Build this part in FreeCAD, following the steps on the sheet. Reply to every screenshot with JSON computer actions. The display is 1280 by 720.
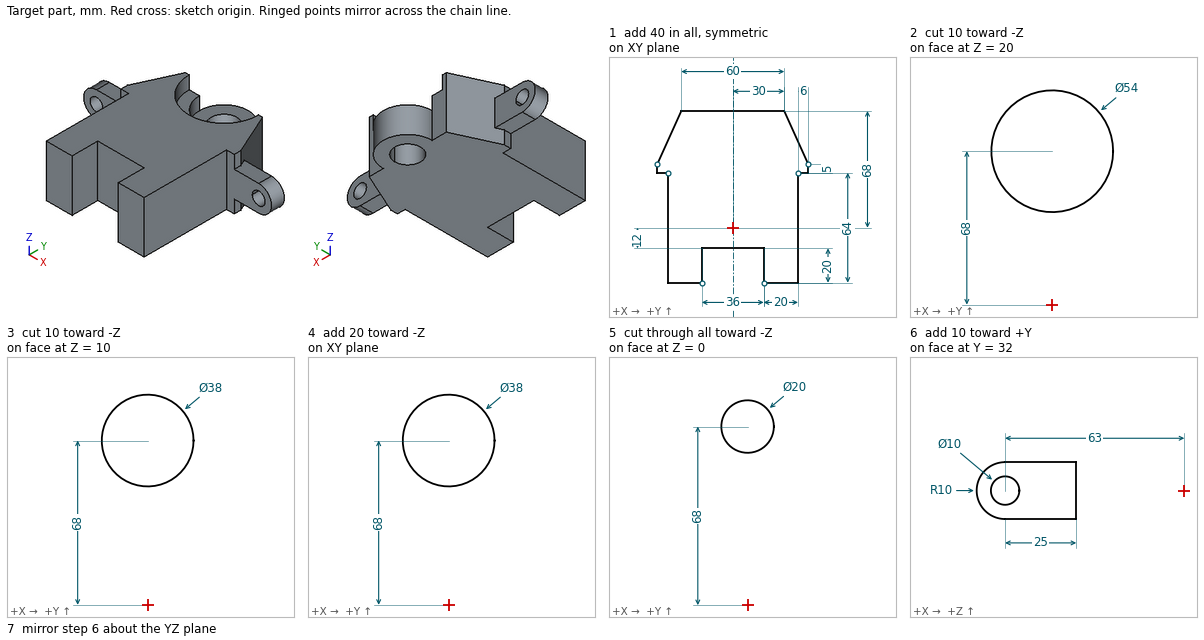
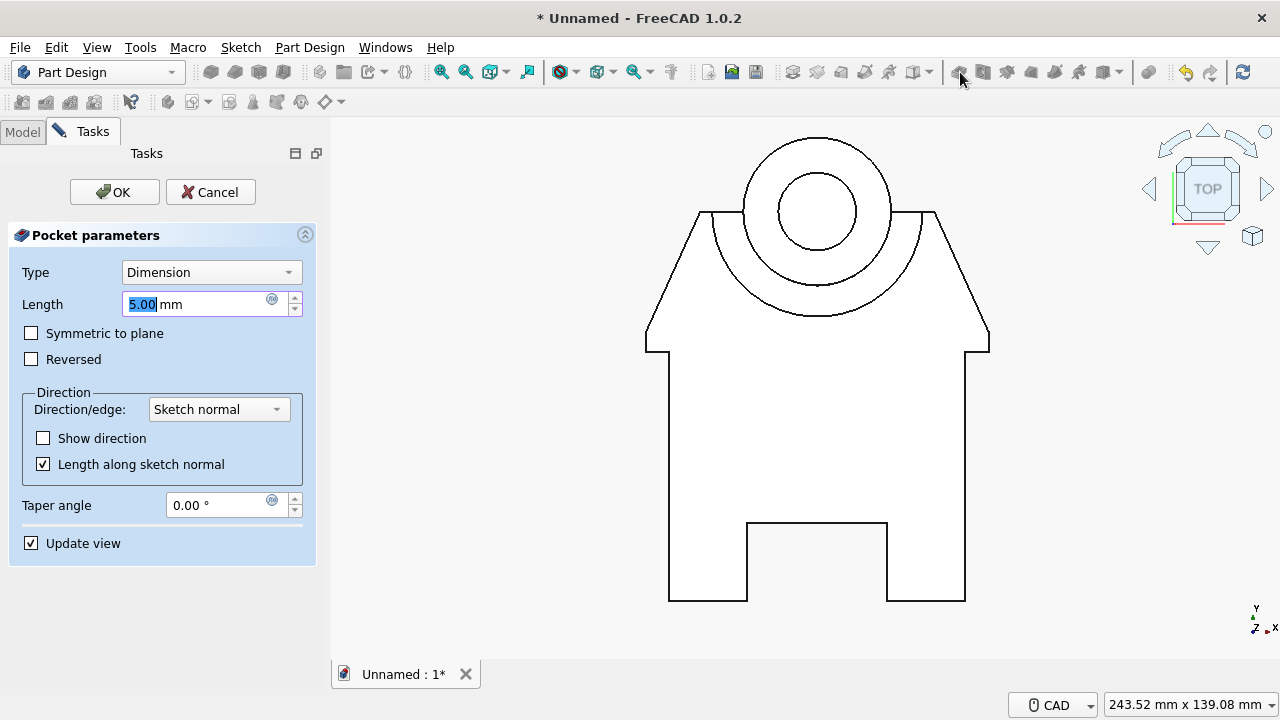
{"action": "left_click", "coordinate": [212, 272]}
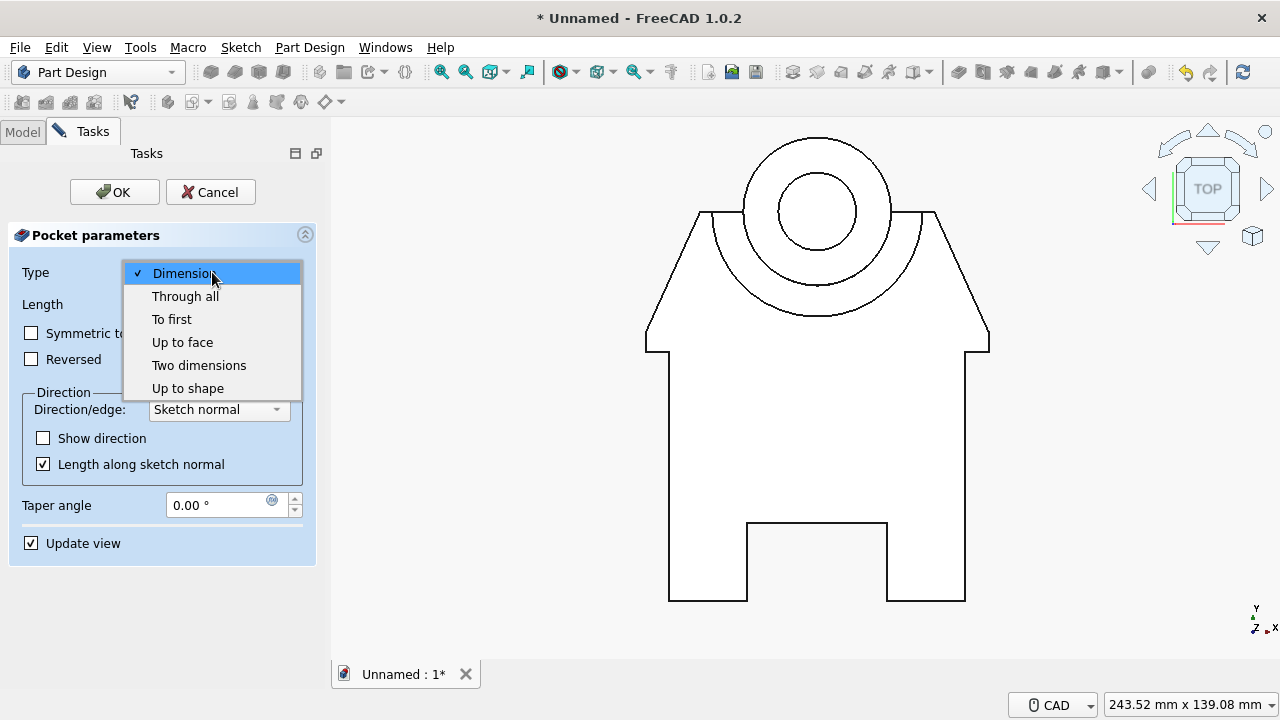
{"action": "left_click", "coordinate": [212, 296]}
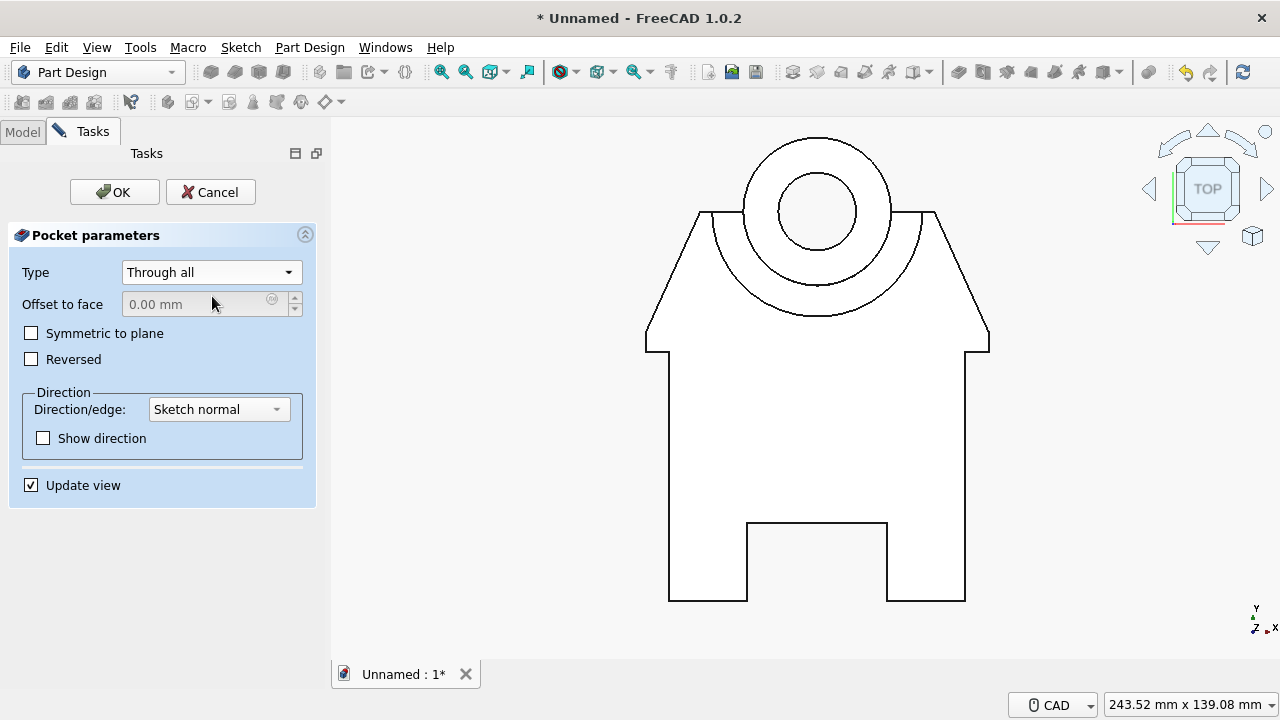
{"action": "left_click", "coordinate": [115, 192]}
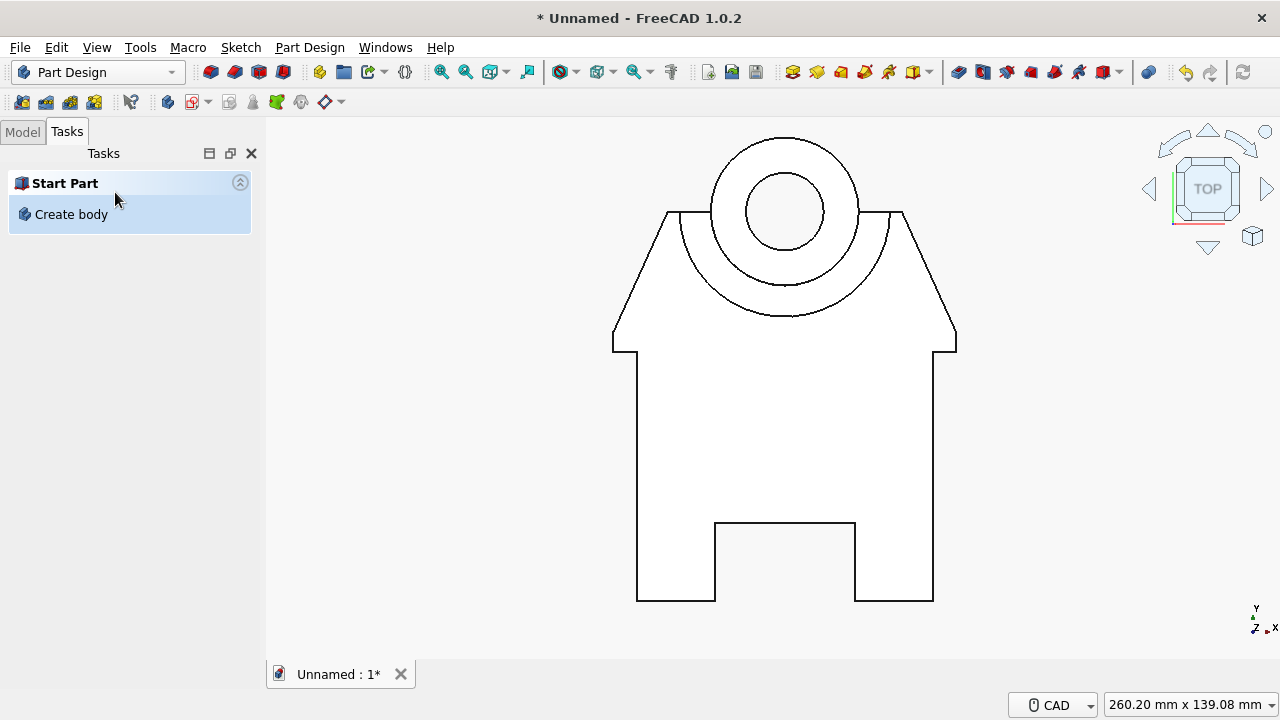
{"action": "key", "text": "0"}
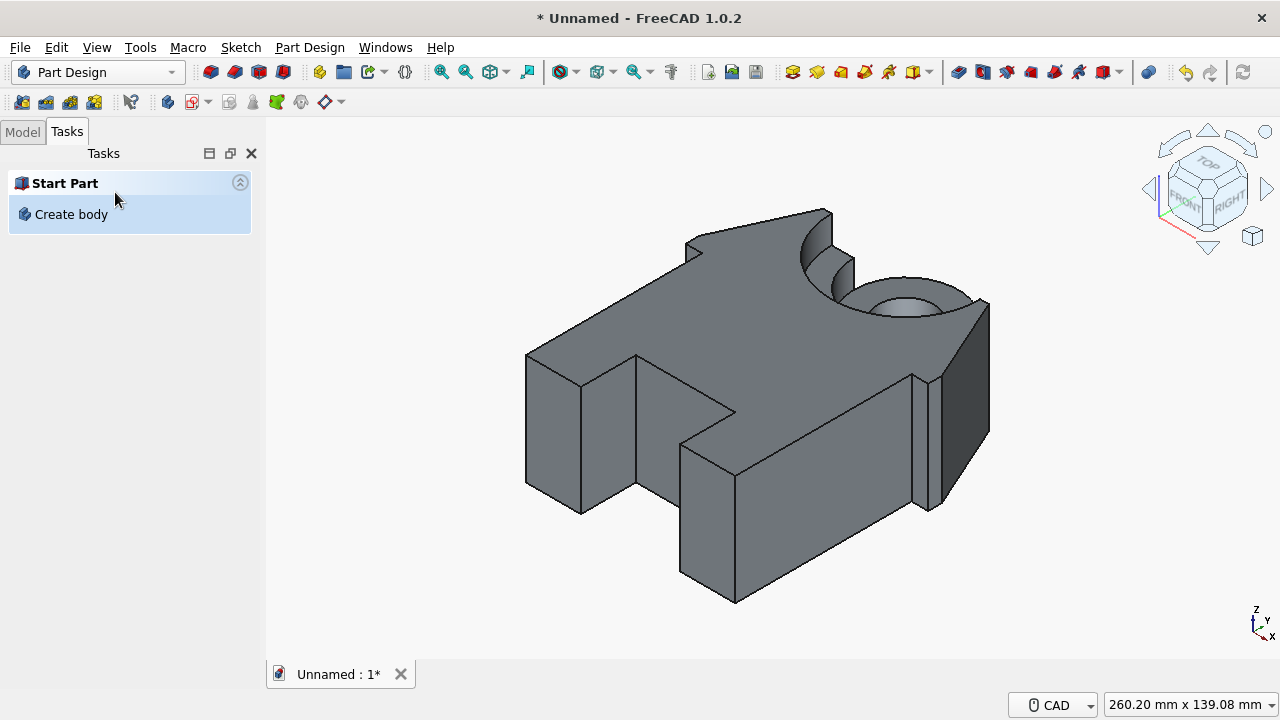
{"action": "key", "text": "1"}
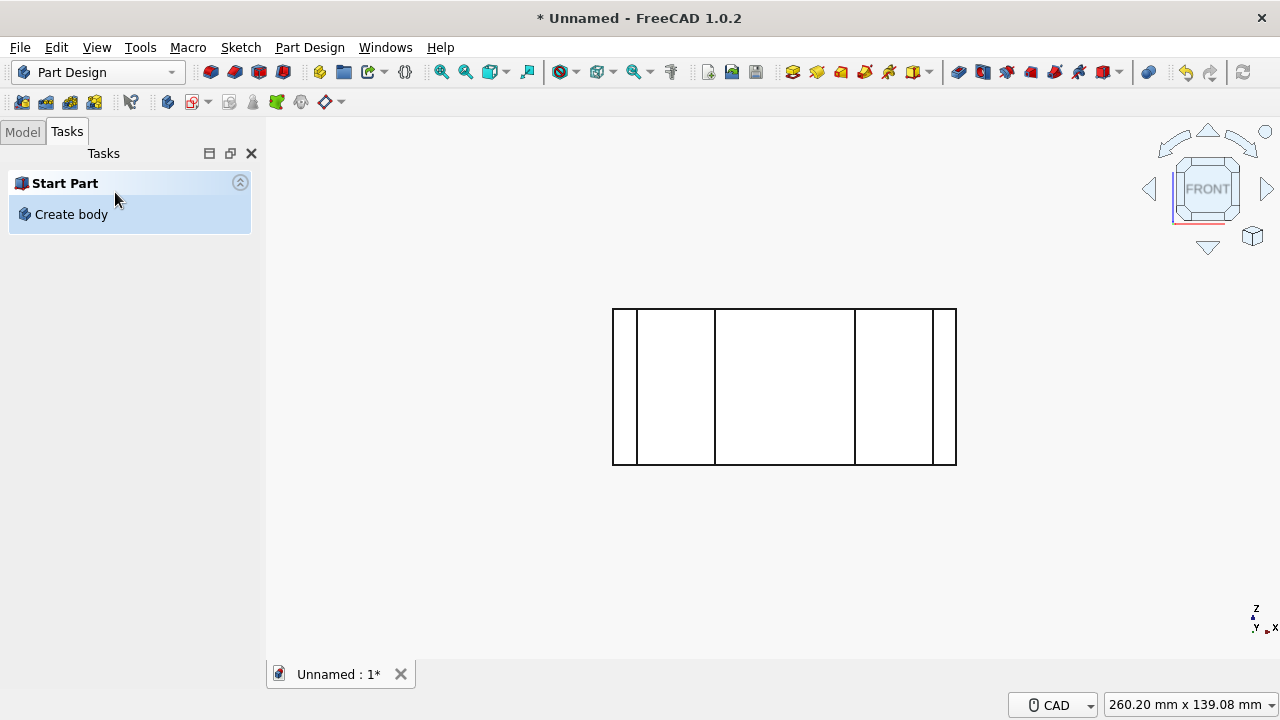
{"action": "left_click", "coordinate": [442, 72]}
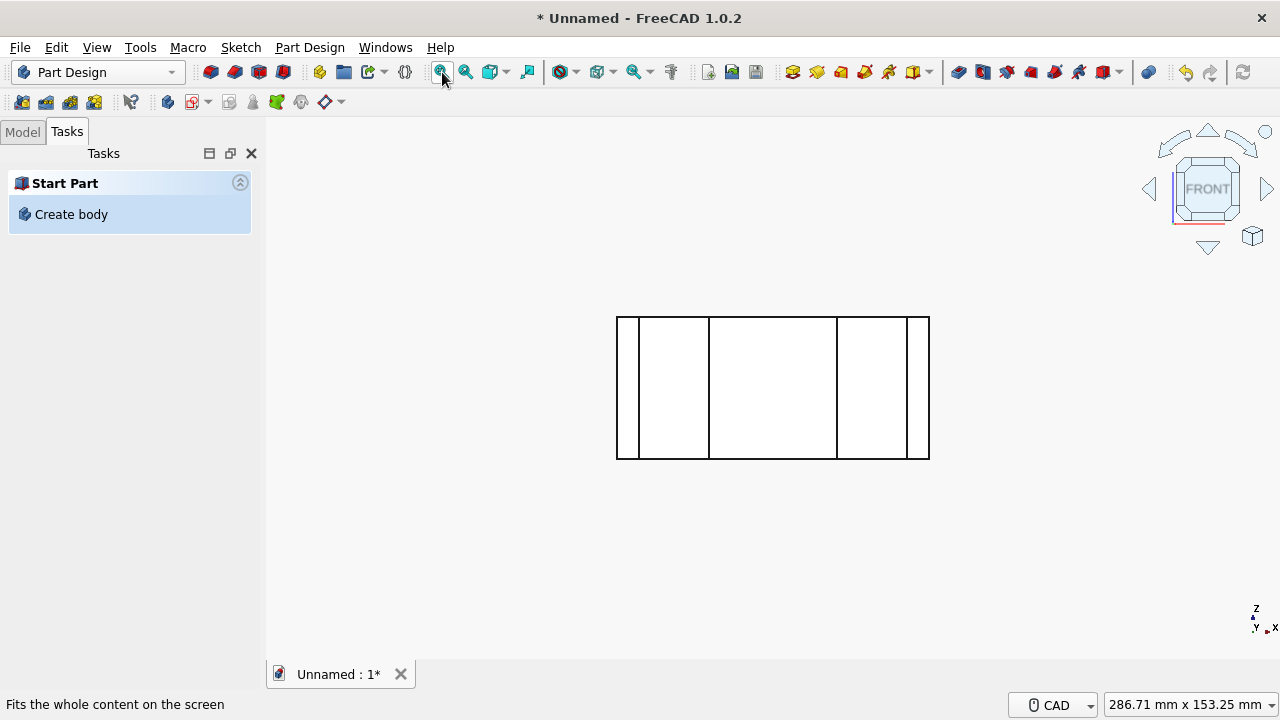
{"action": "left_click", "coordinate": [628, 347]}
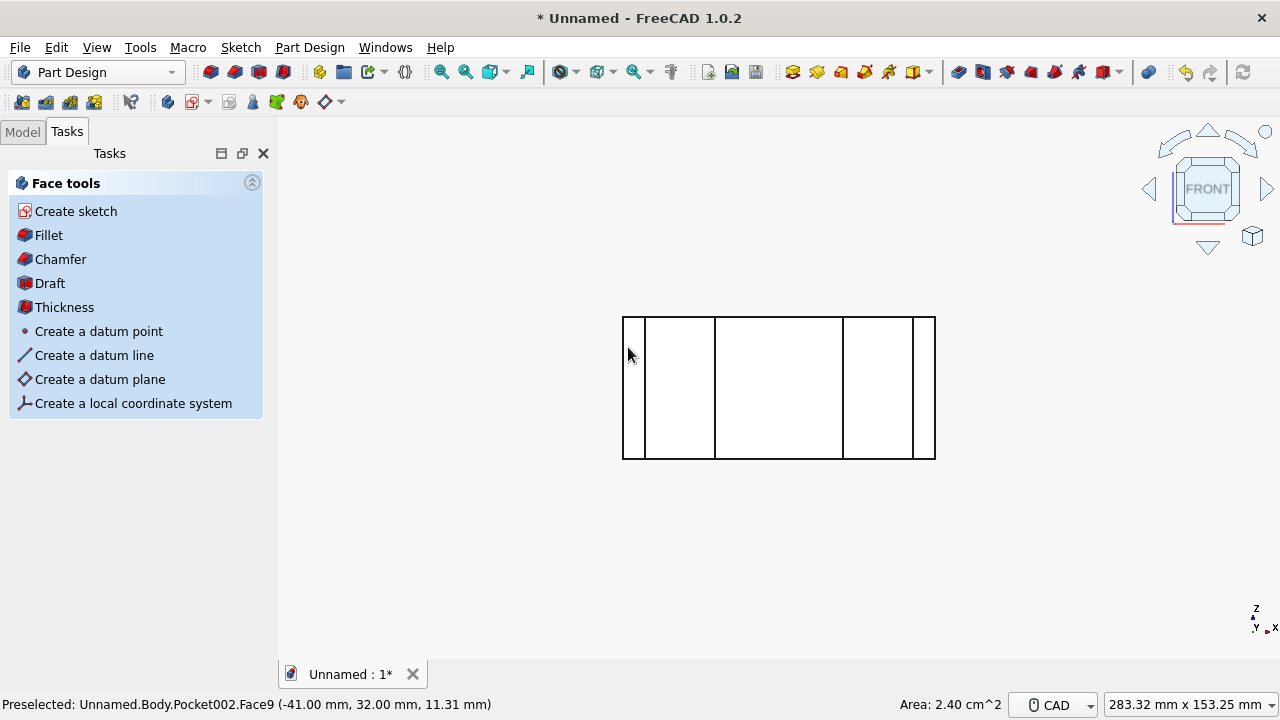
{"action": "left_click", "coordinate": [192, 102]}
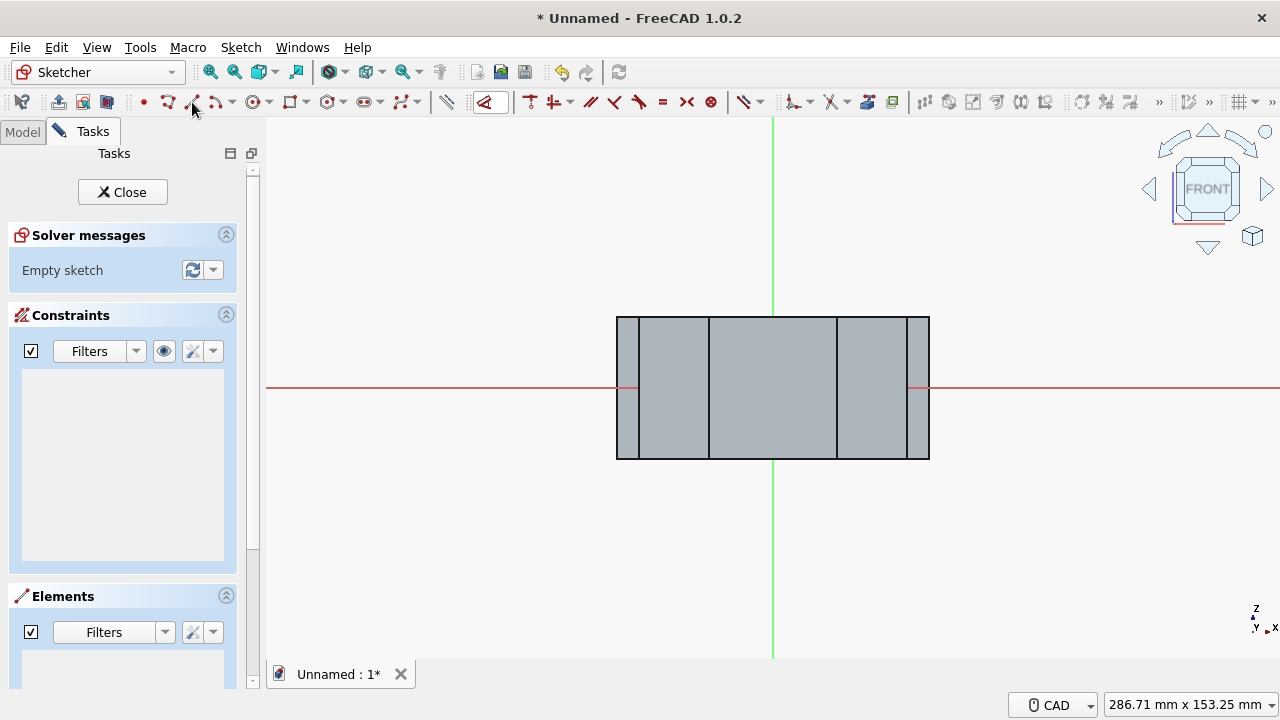
{"action": "scroll", "coordinate": [594, 388], "scroll_direction": "up", "scroll_amount": 4}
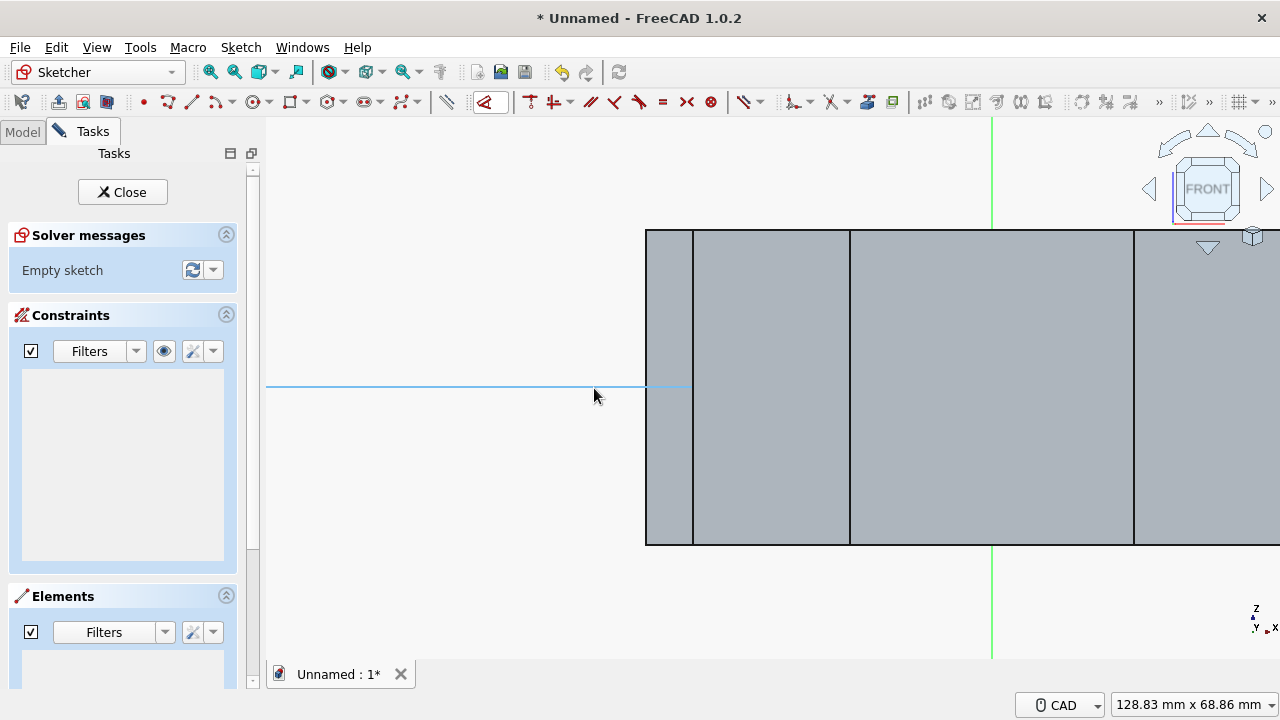
{"action": "left_click", "coordinate": [168, 102]}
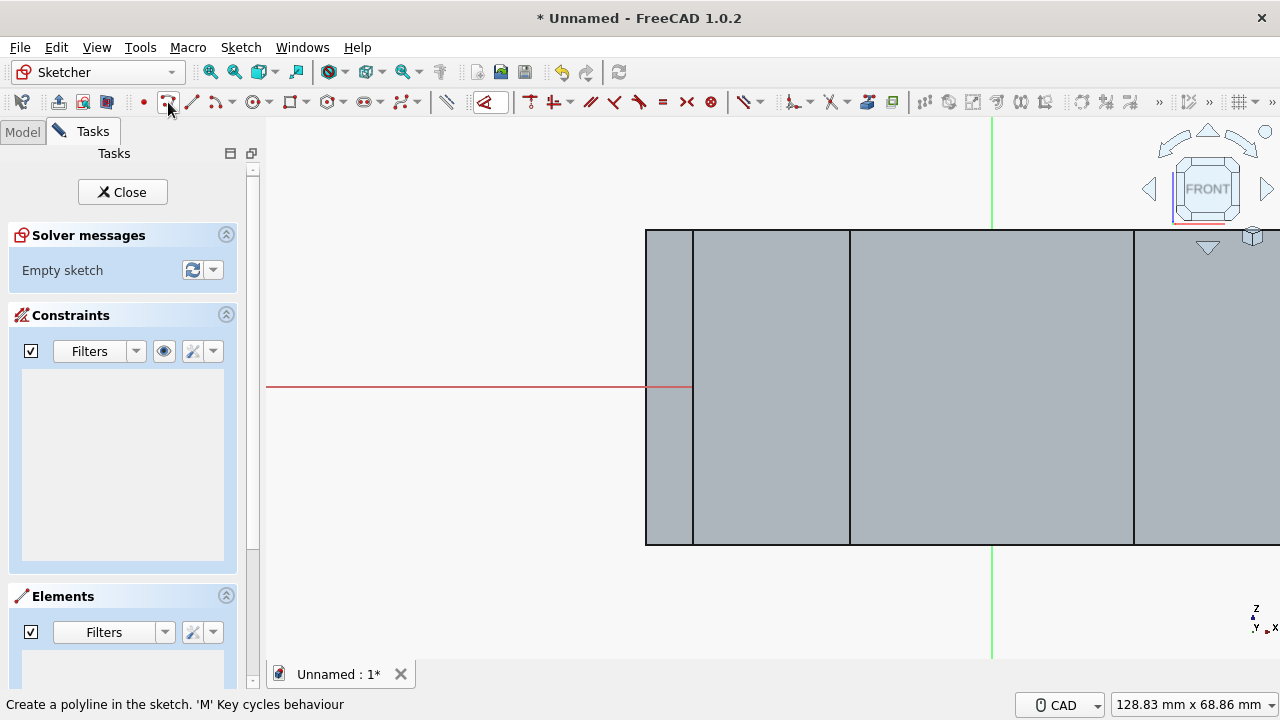
{"action": "left_click", "coordinate": [496, 466]}
{"action": "left_click", "coordinate": [693, 466]}
{"action": "left_click", "coordinate": [693, 309]}
{"action": "left_click", "coordinate": [496, 309]}
{"action": "right_click", "coordinate": [496, 309]}